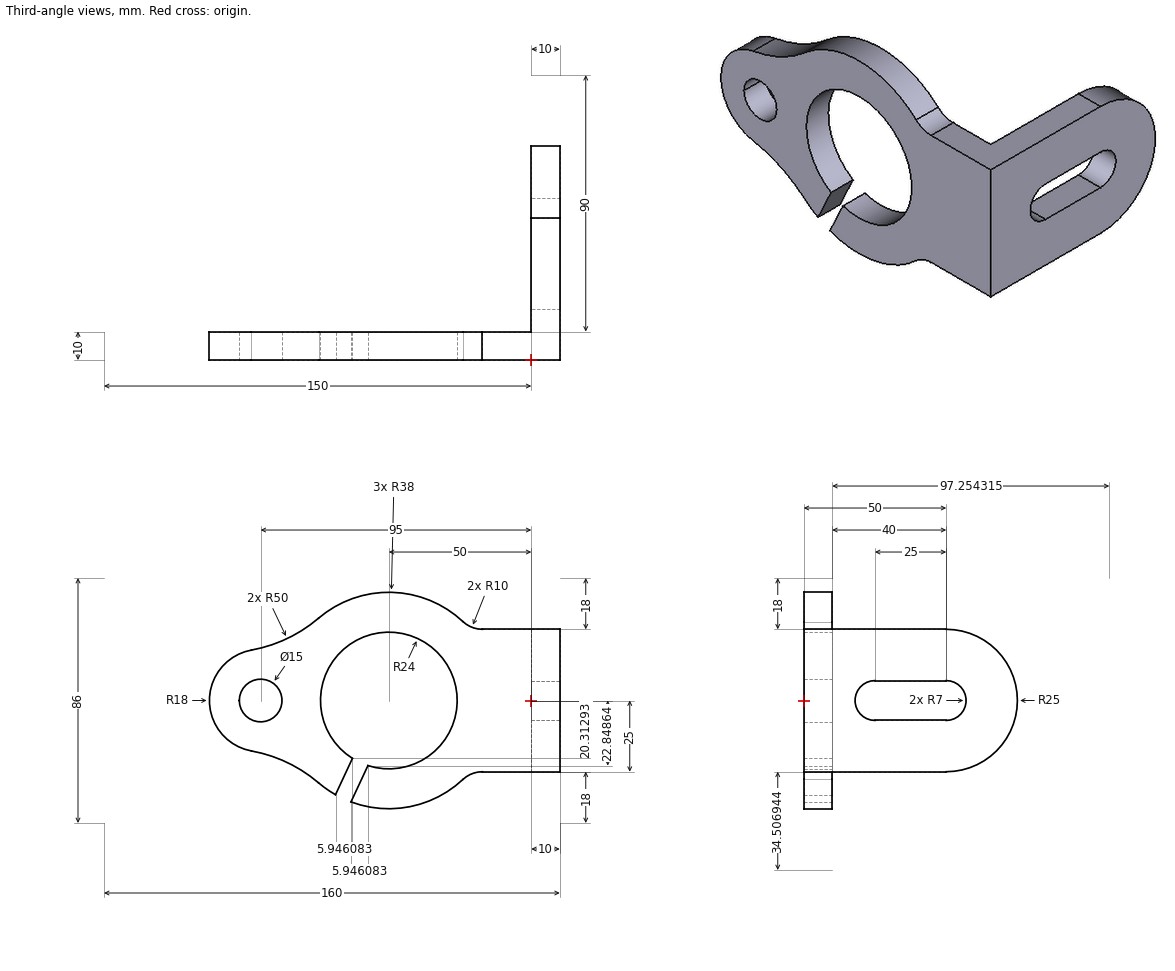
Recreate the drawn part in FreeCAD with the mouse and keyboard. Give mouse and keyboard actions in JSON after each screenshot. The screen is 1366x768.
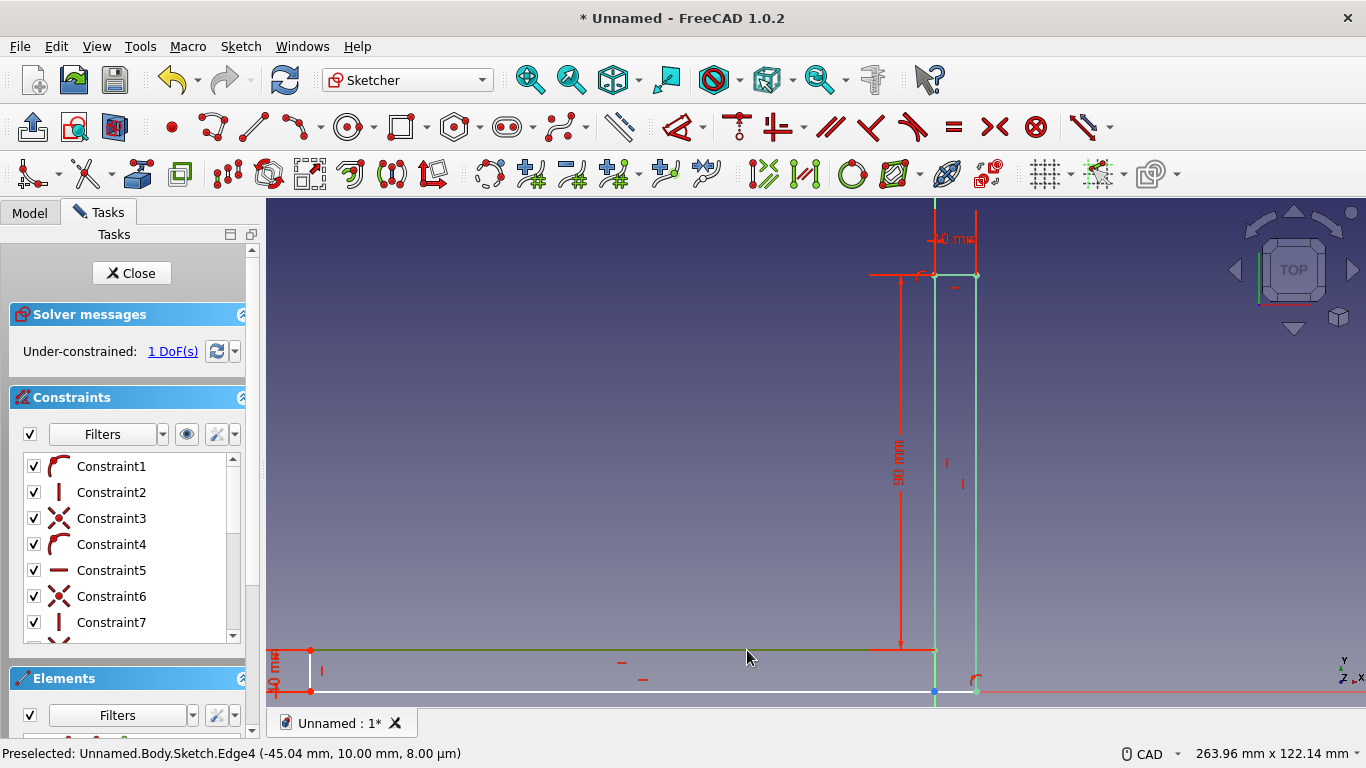
{"action": "key", "text": "l"}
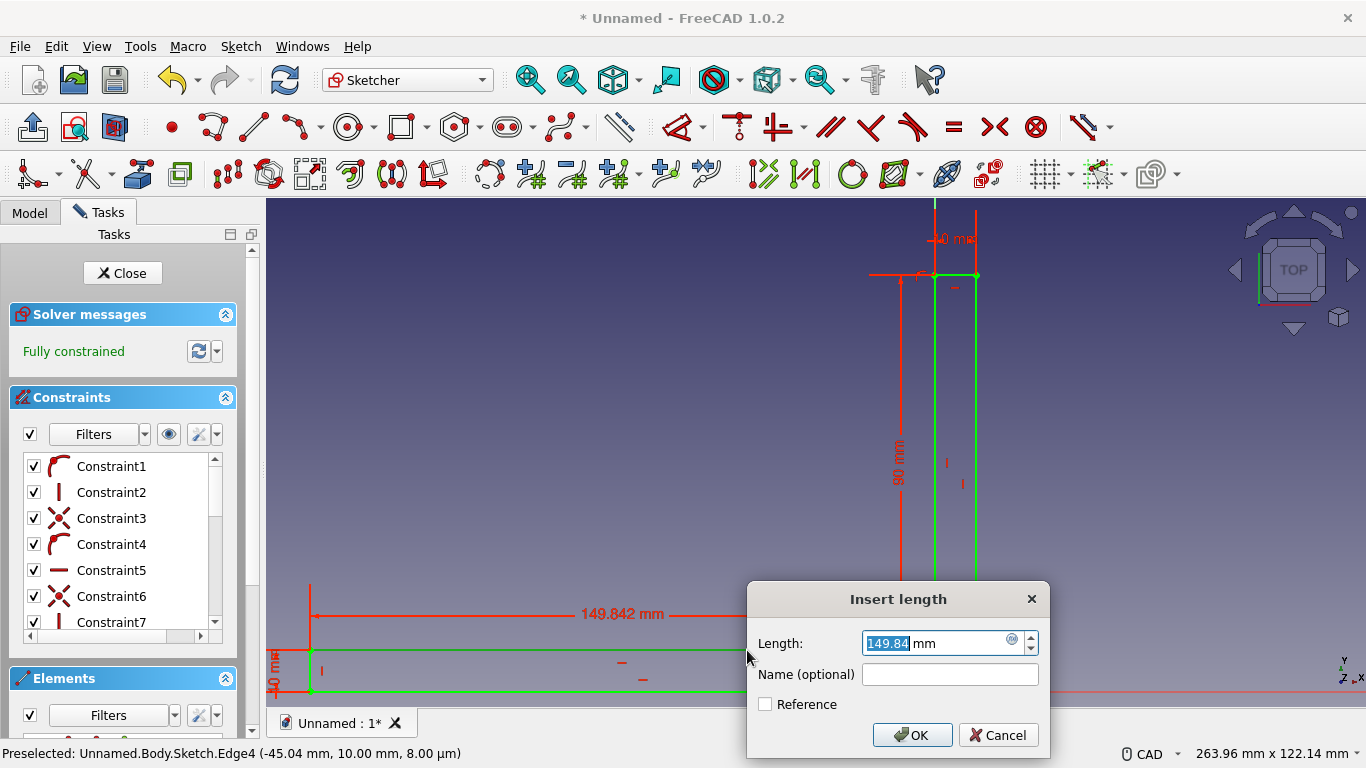
{"action": "type", "text": "150"}
{"action": "key", "text": "Return"}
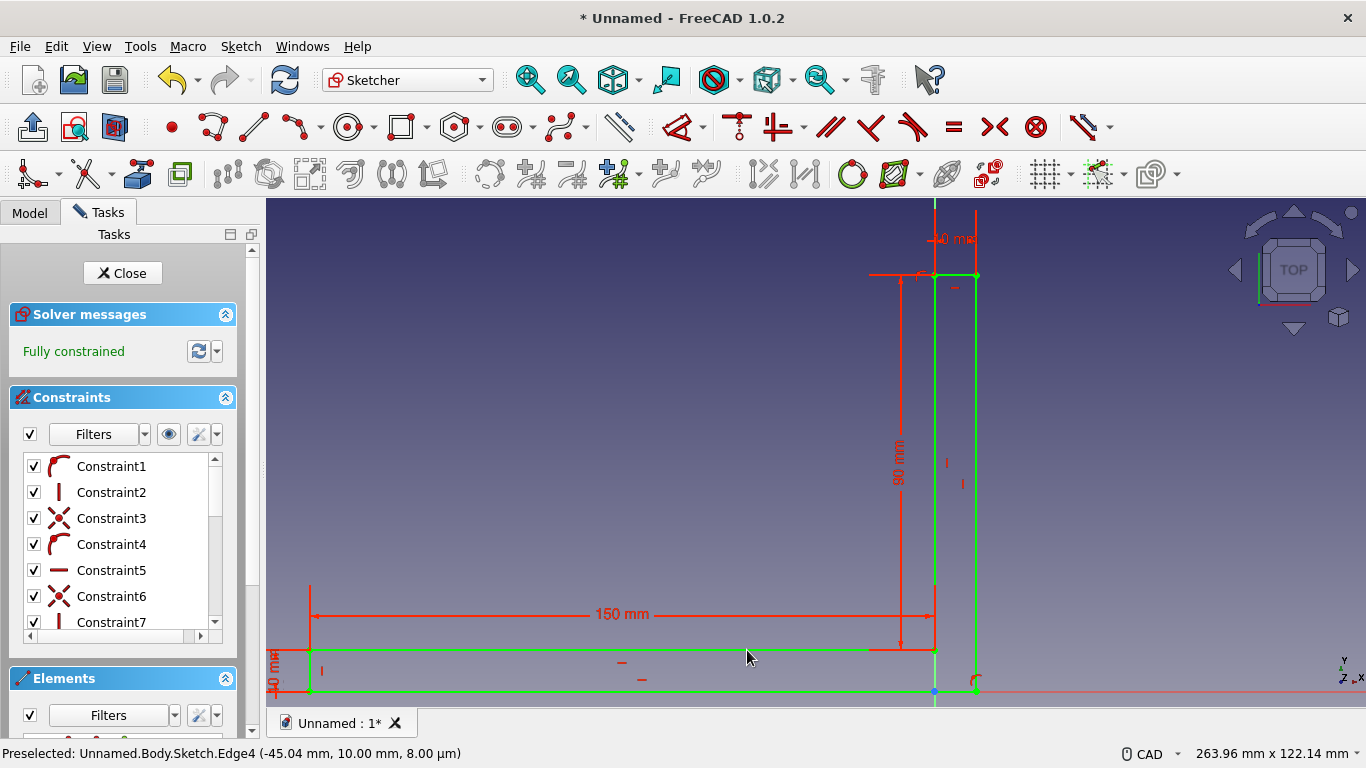
{"action": "left_click", "coordinate": [123, 273]}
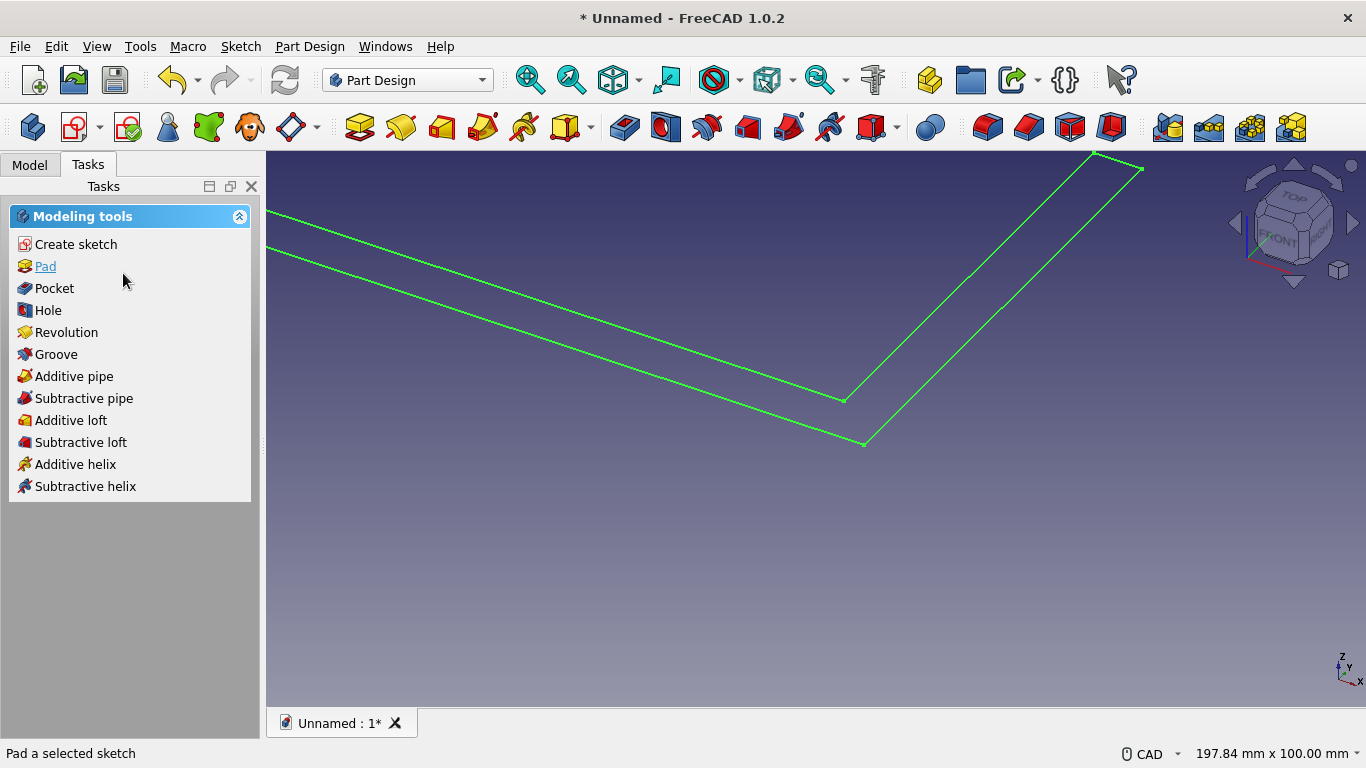
{"action": "left_click", "coordinate": [360, 128]}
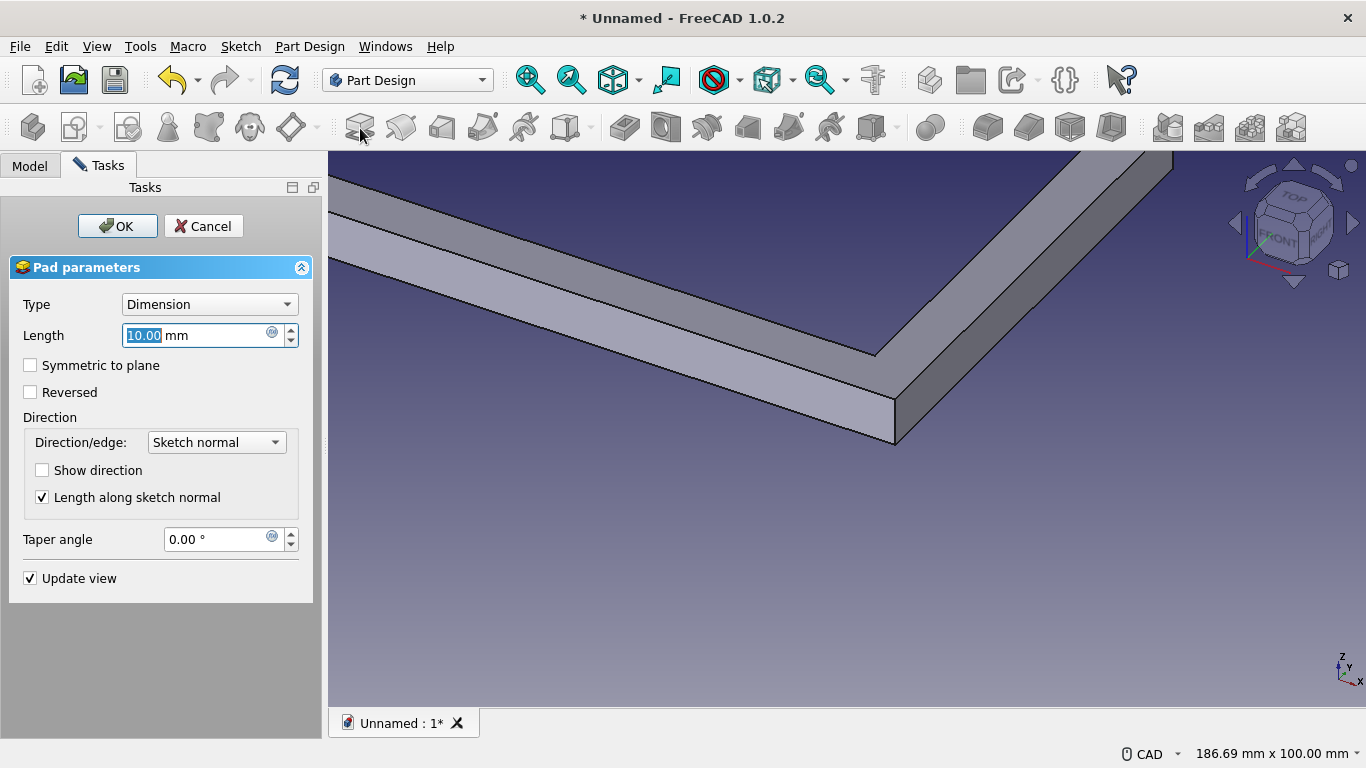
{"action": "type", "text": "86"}
{"action": "key", "text": "Tab"}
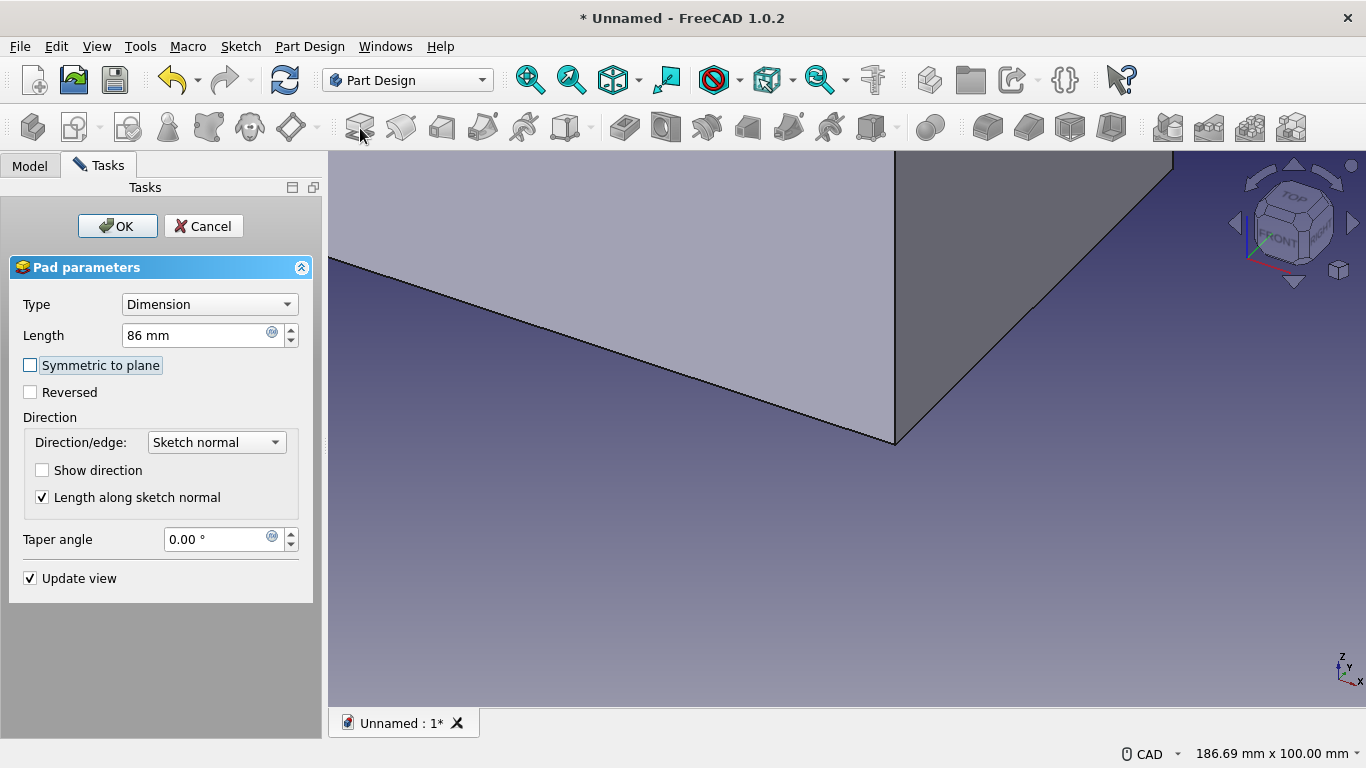
{"action": "left_click", "coordinate": [31, 365]}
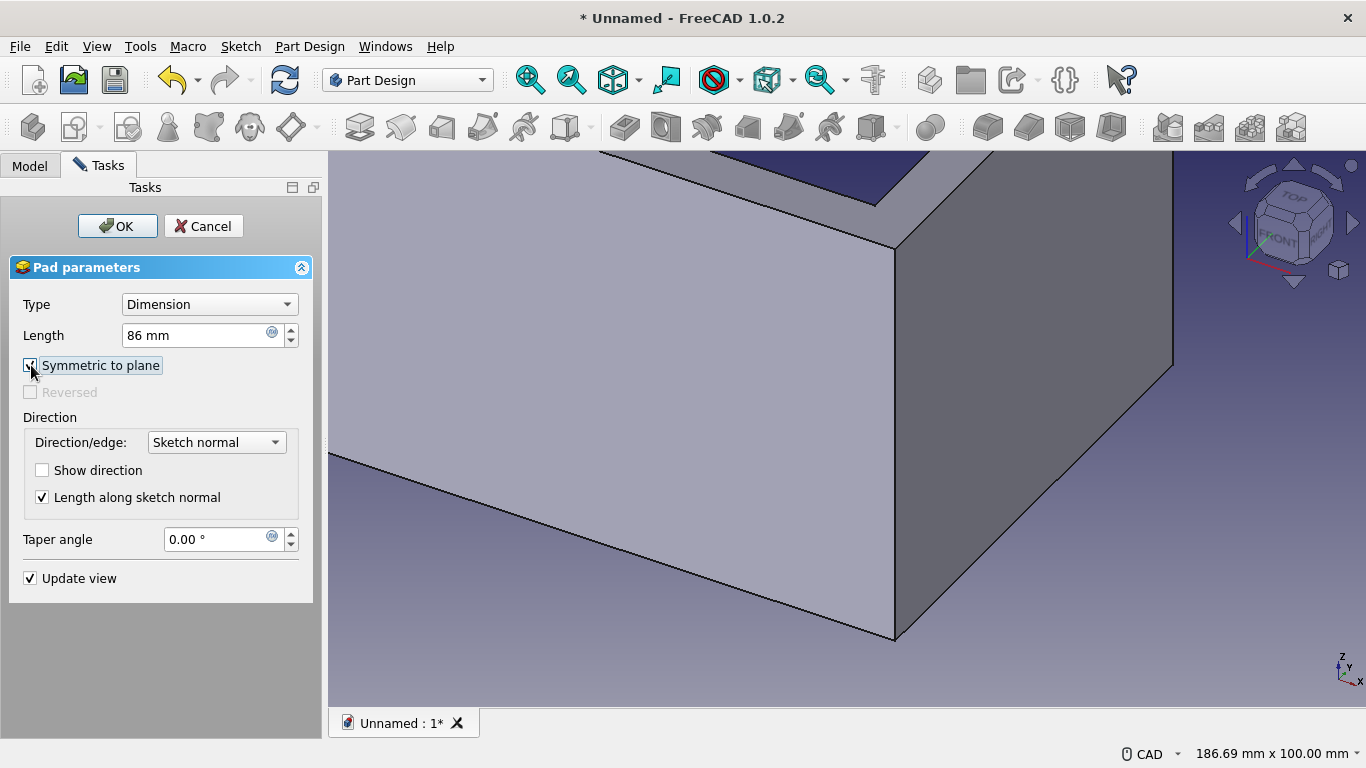
{"action": "left_click", "coordinate": [118, 226]}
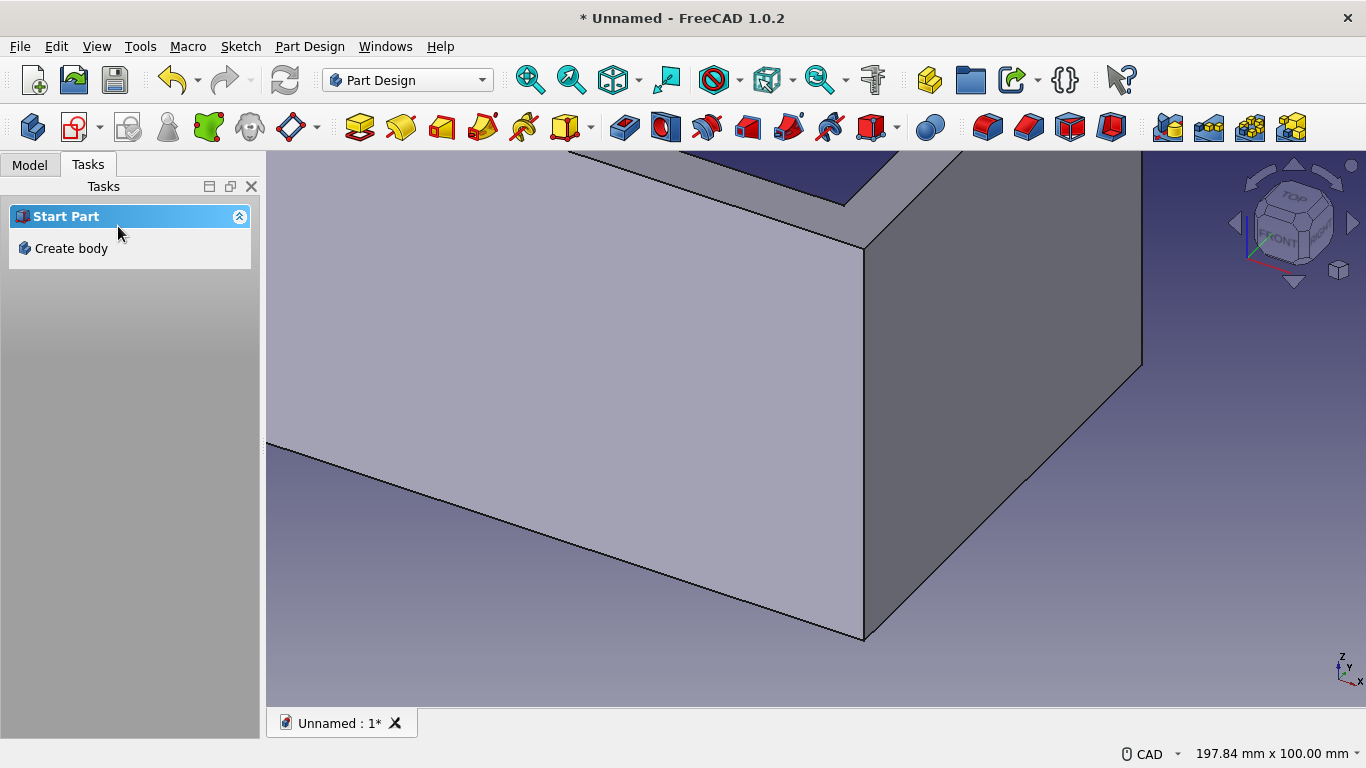
{"action": "left_click", "coordinate": [531, 80]}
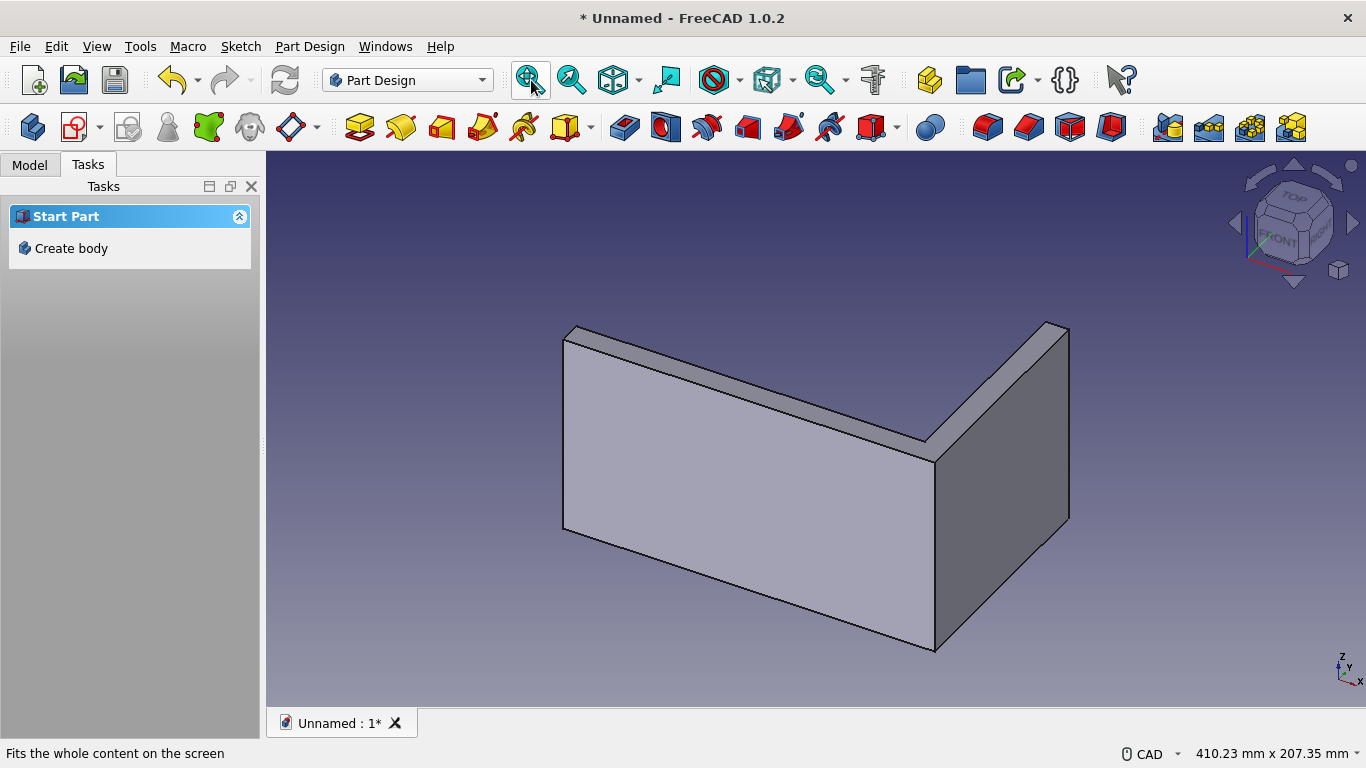
{"action": "key", "text": "6"}